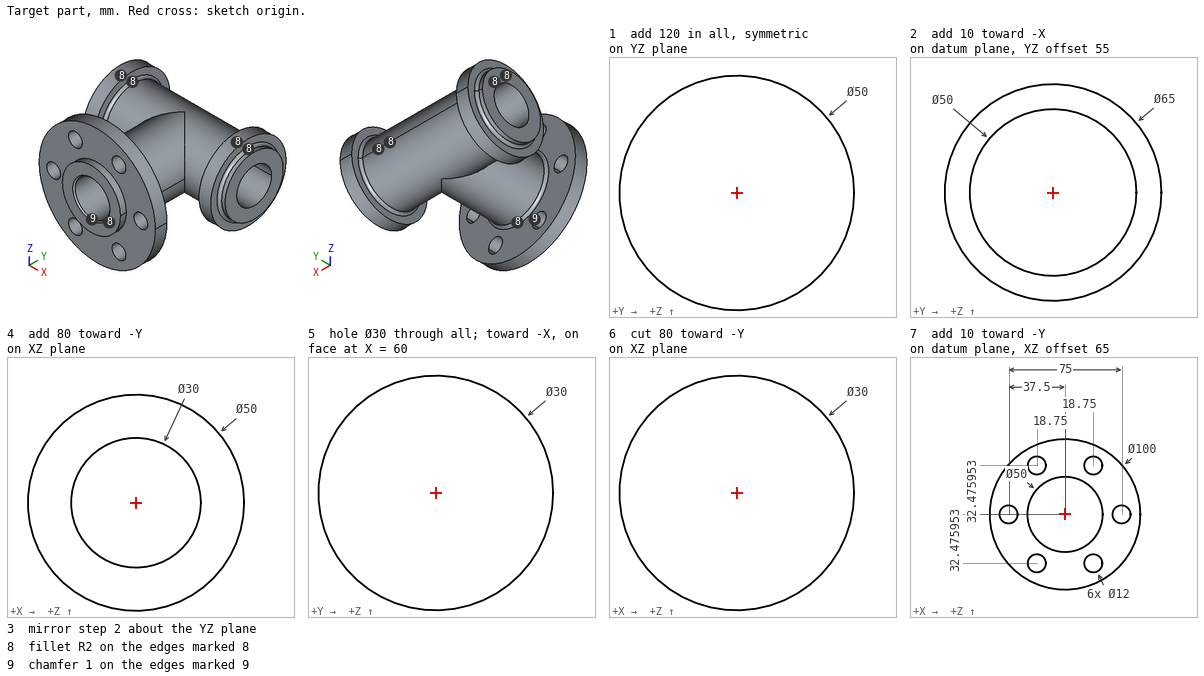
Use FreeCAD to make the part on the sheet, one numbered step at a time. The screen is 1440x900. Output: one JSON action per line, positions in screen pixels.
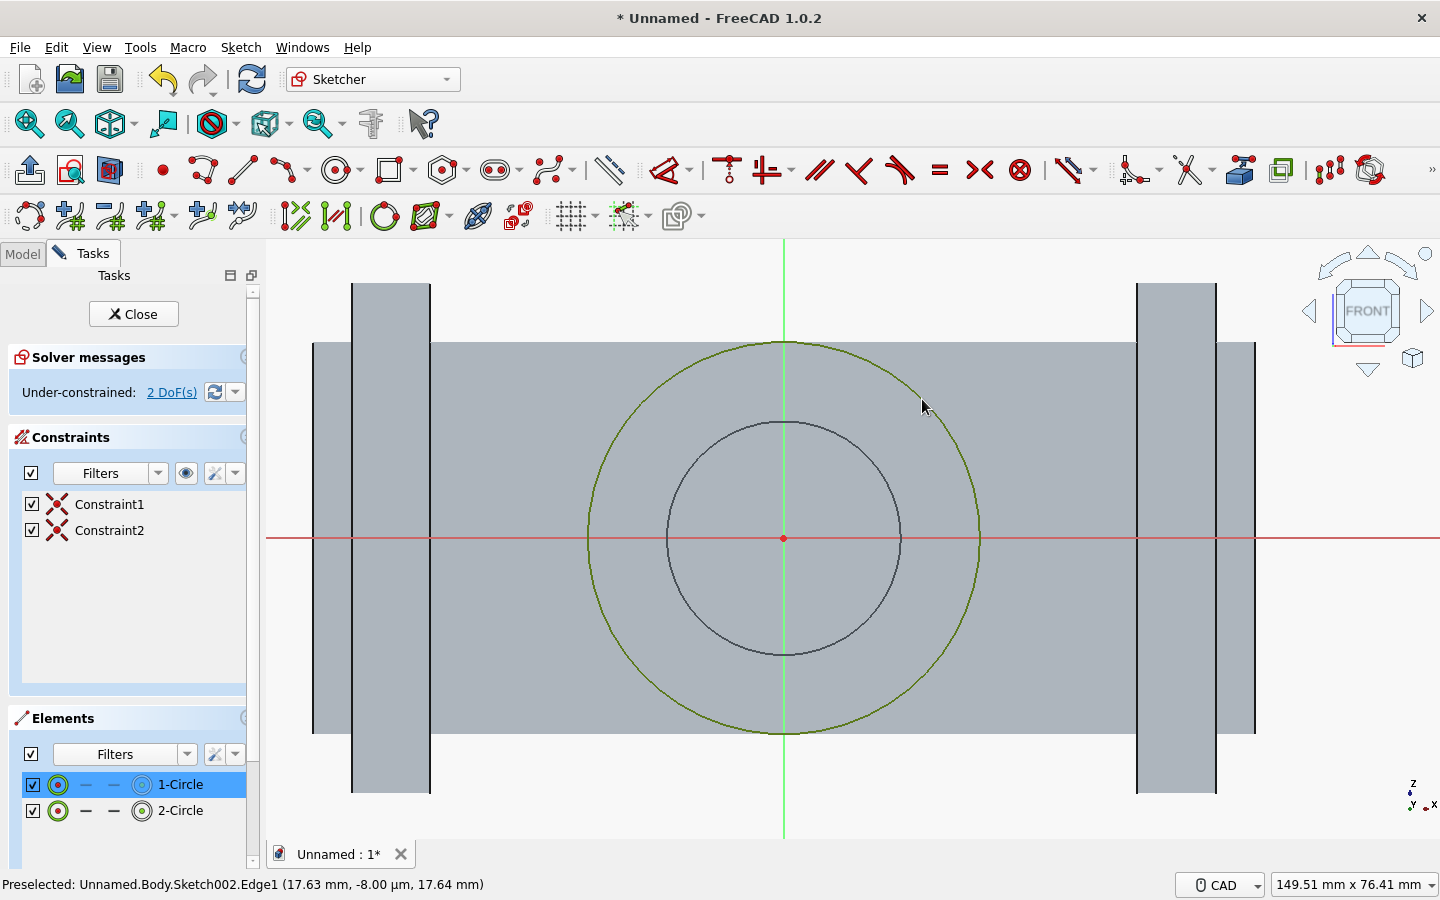
{"action": "key", "text": "k o"}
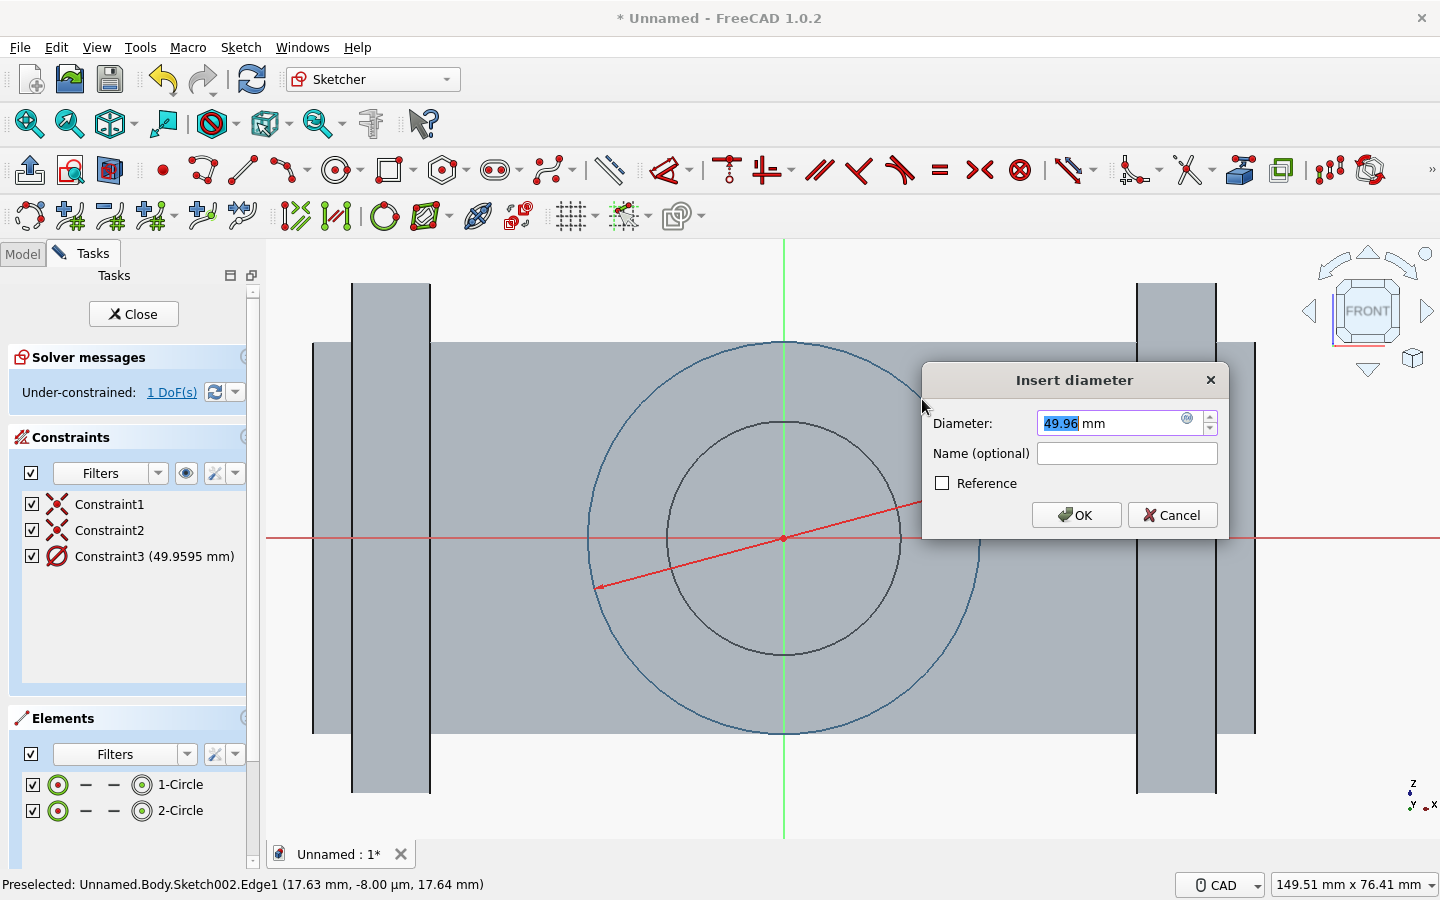
{"action": "type", "text": "50"}
{"action": "key", "text": "Return"}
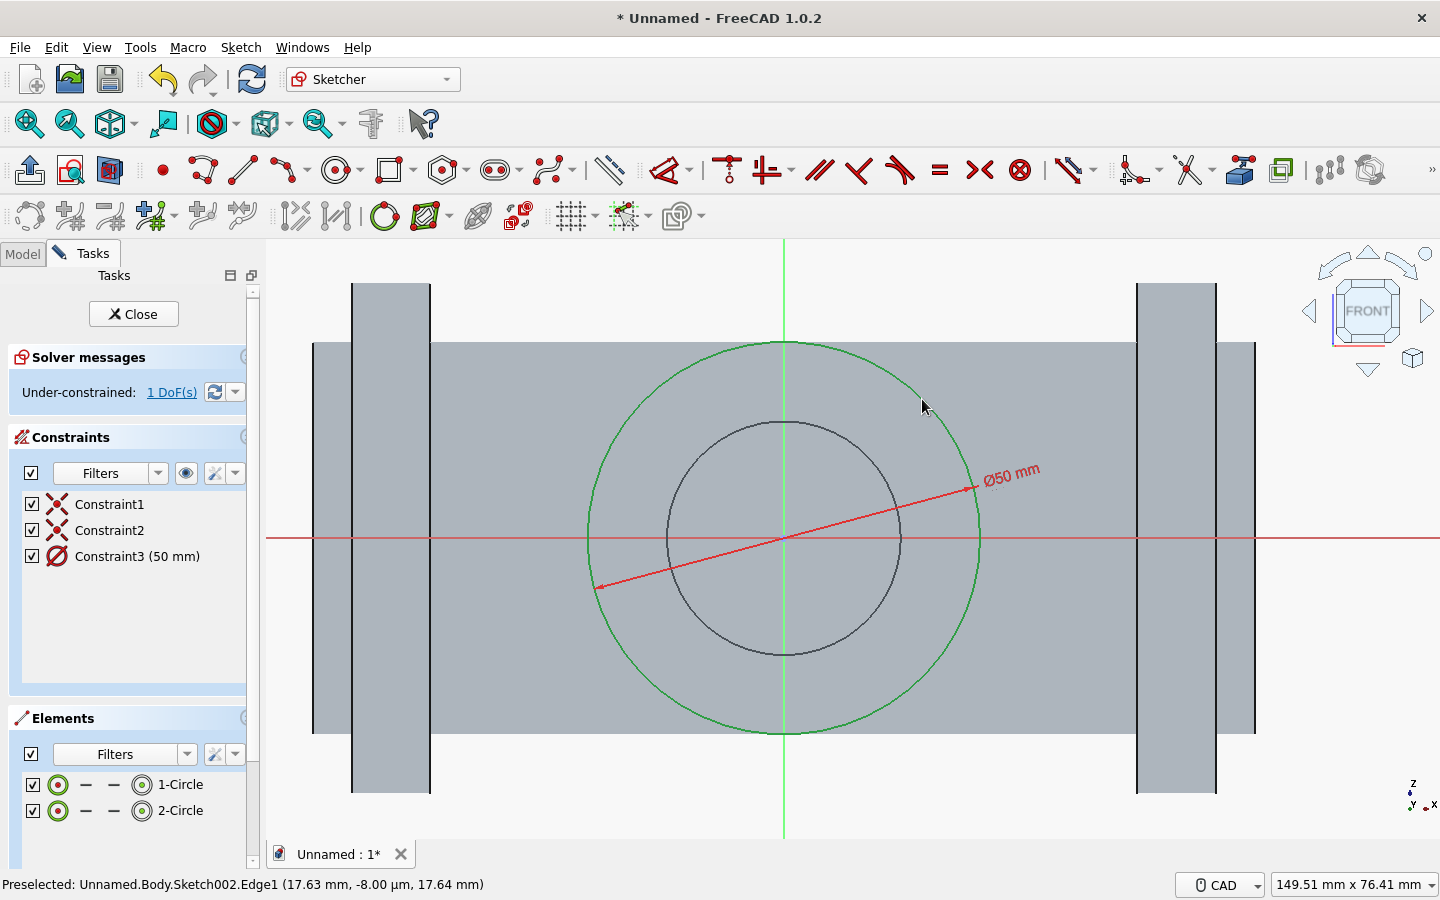
{"action": "left_click", "coordinate": [866, 455]}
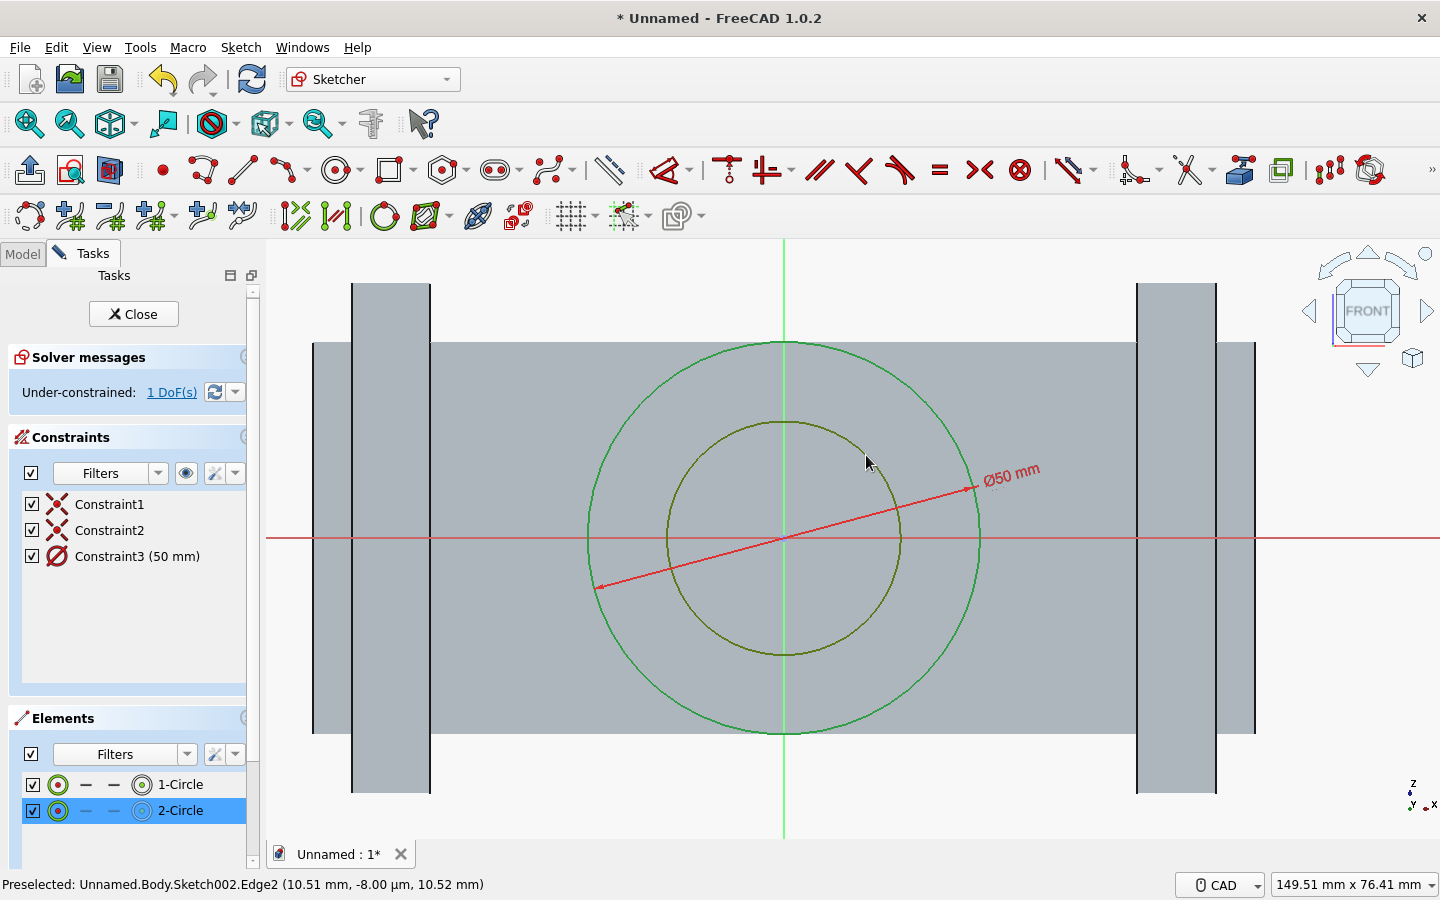
{"action": "key", "text": "k o"}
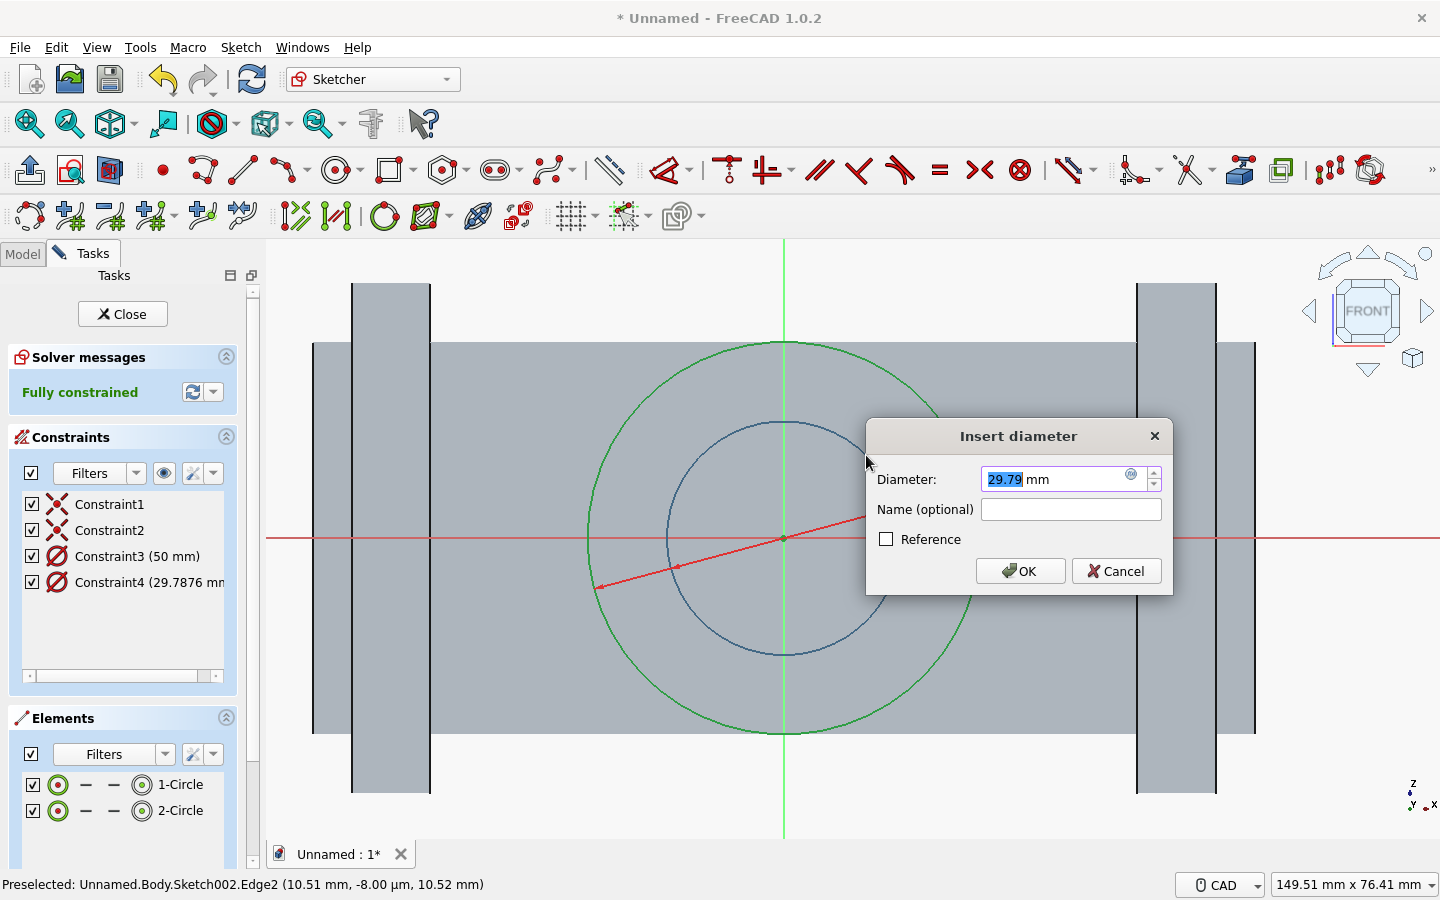
{"action": "type", "text": "30"}
{"action": "key", "text": "Return"}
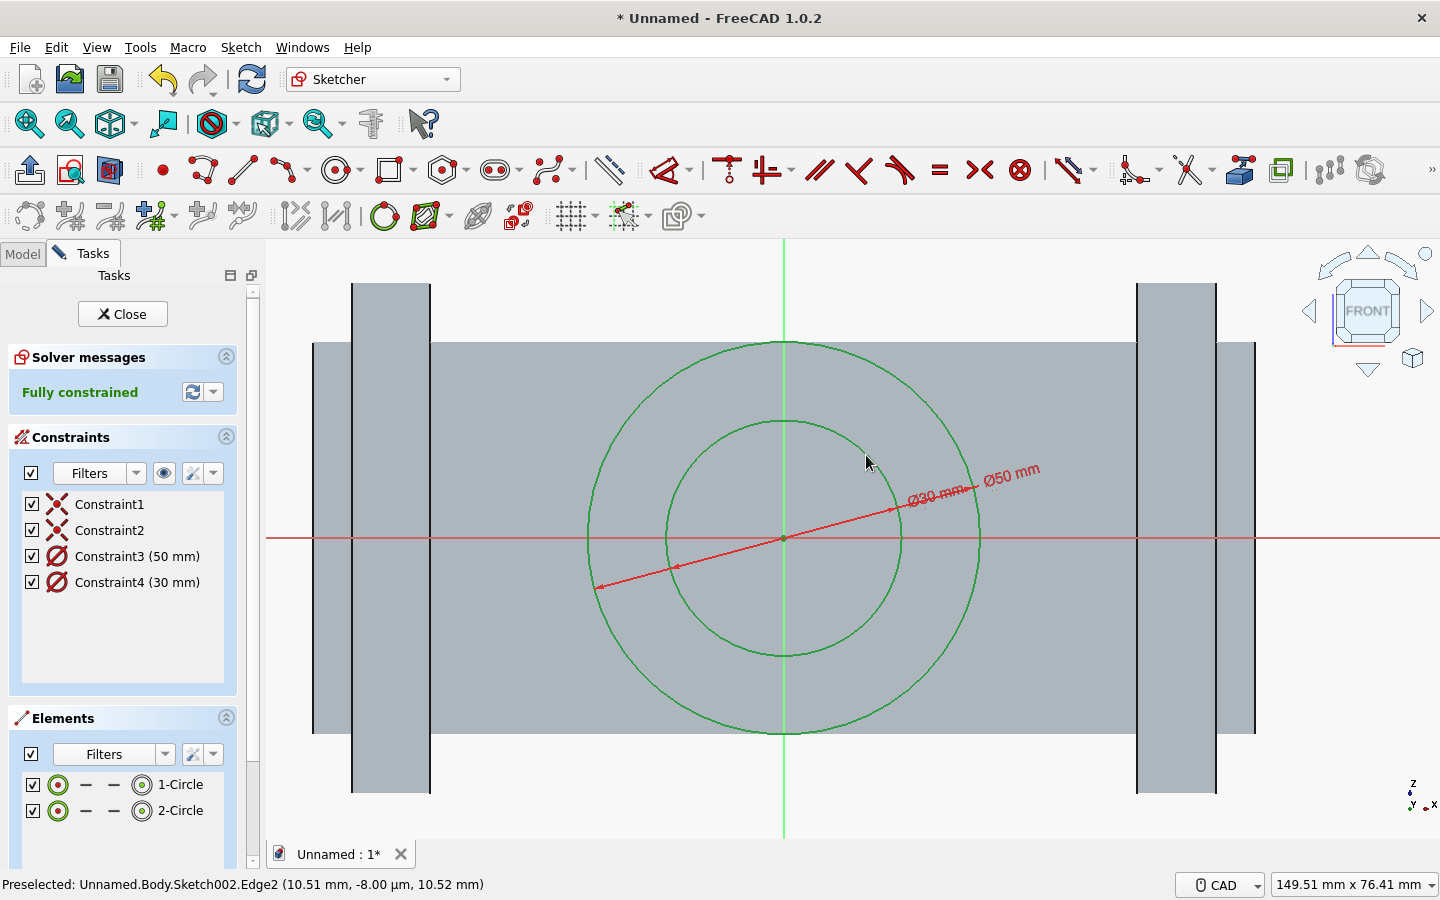
{"action": "left_click", "coordinate": [123, 314]}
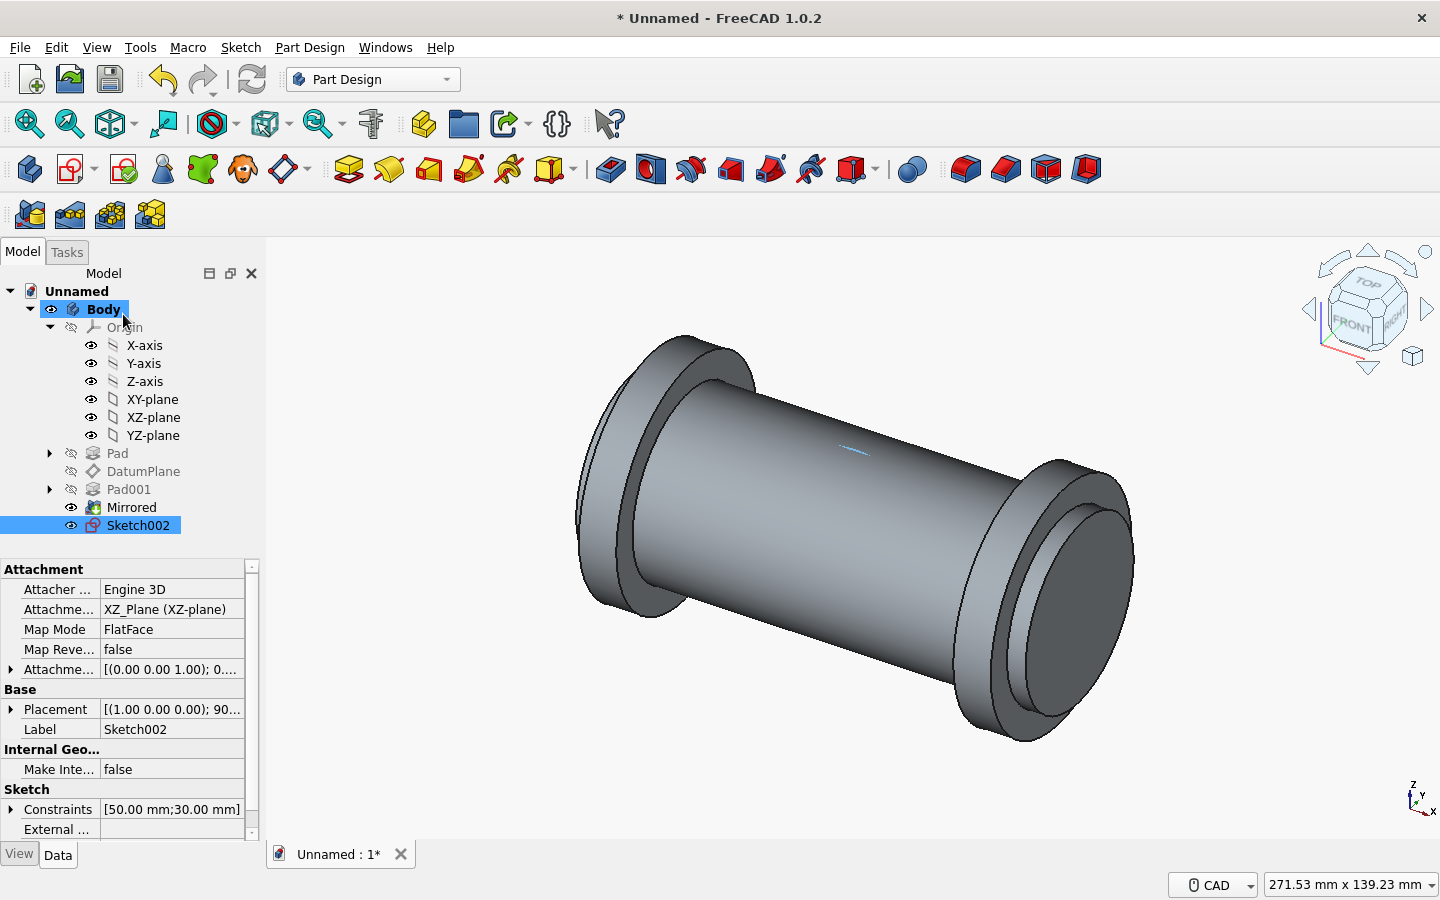
{"action": "left_click", "coordinate": [350, 170]}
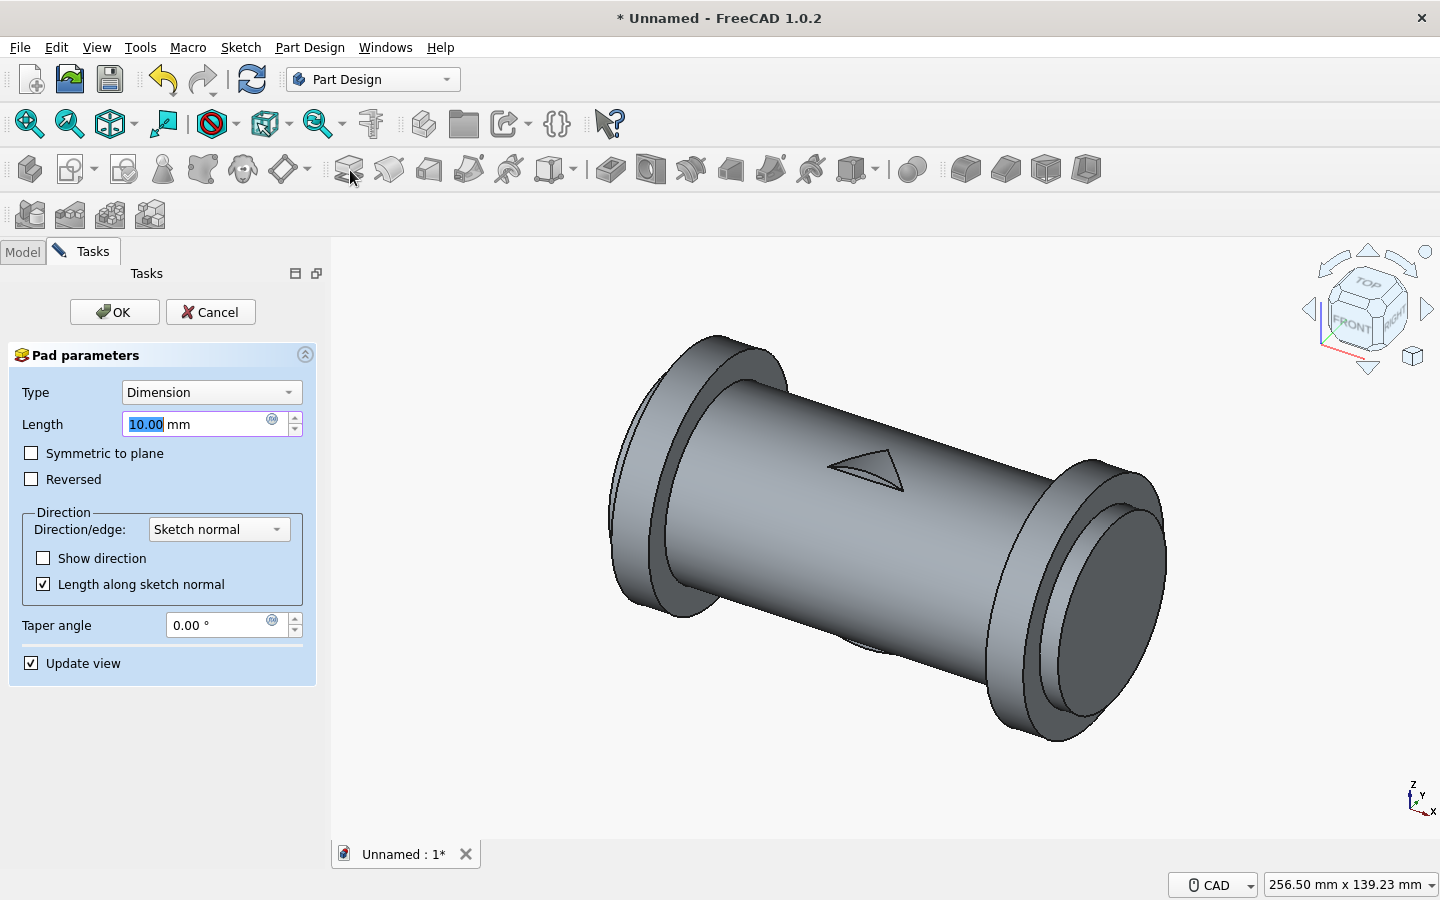
{"action": "type", "text": "80"}
{"action": "key", "text": "Tab"}